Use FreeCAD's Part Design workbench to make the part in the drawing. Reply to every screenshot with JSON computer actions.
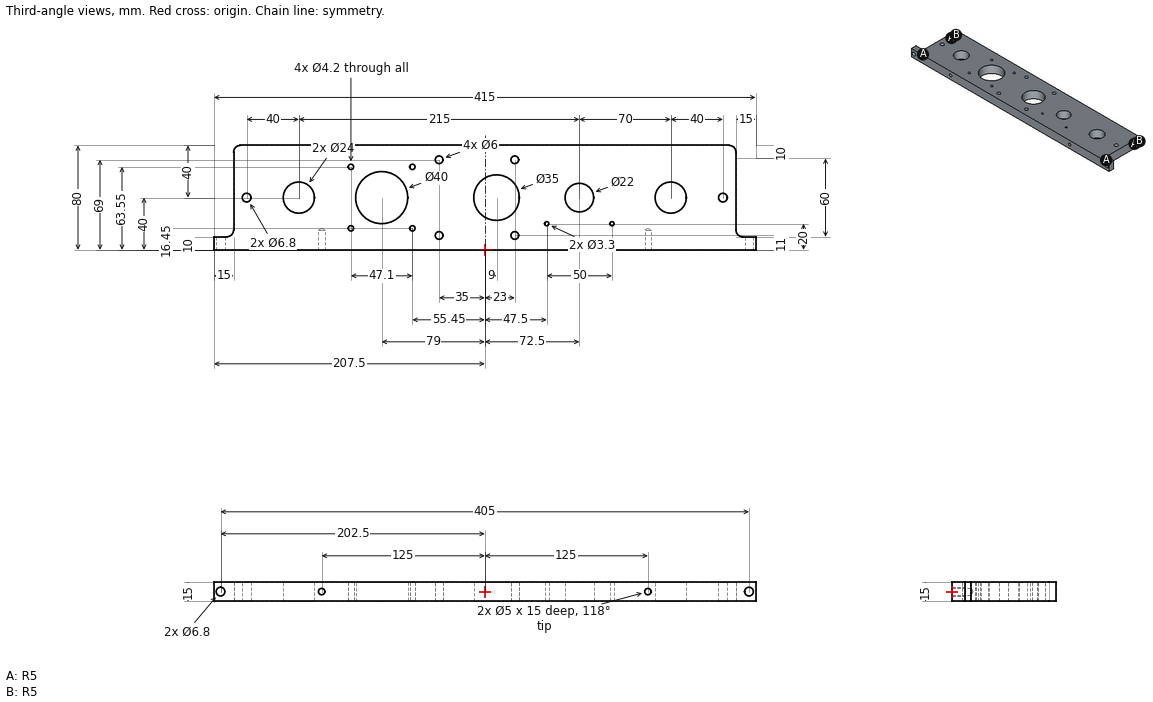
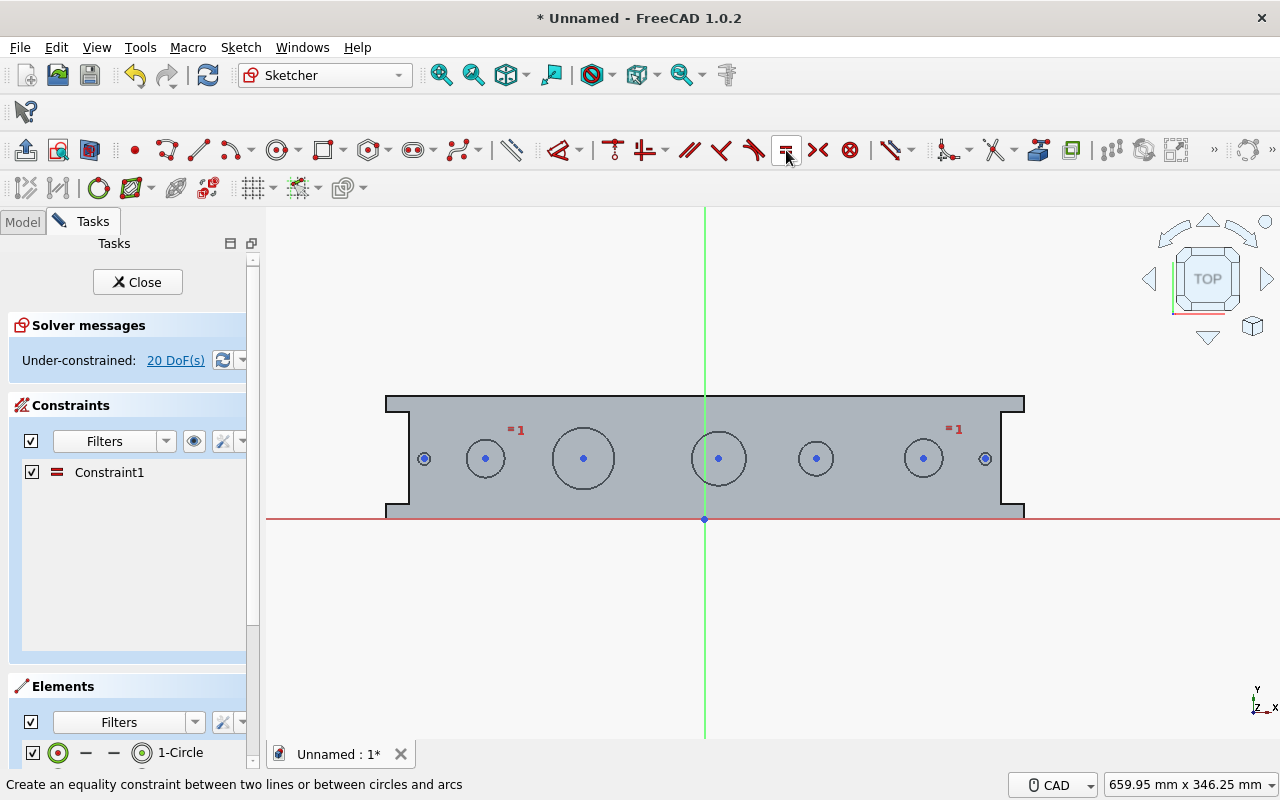
{"action": "scroll", "coordinate": [424, 453], "scroll_direction": "up", "scroll_amount": 5}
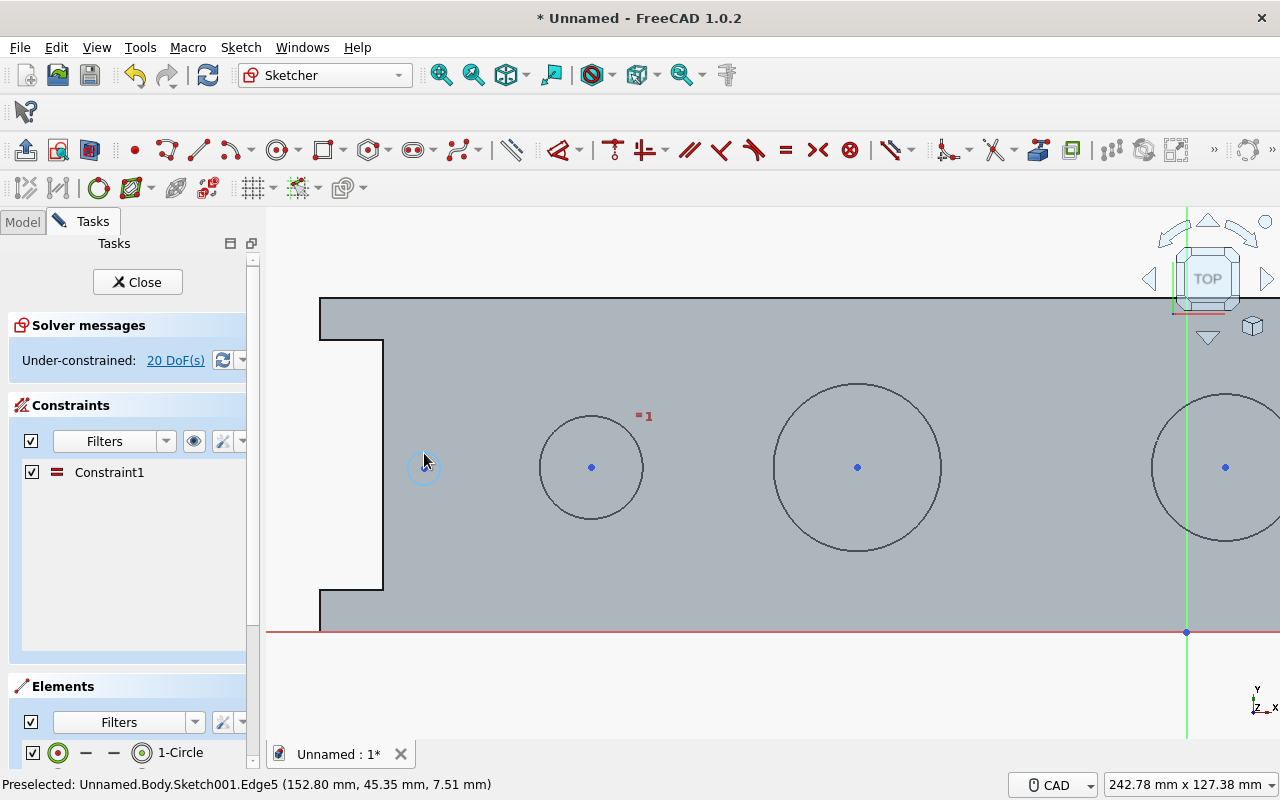
{"action": "left_click", "coordinate": [424, 452]}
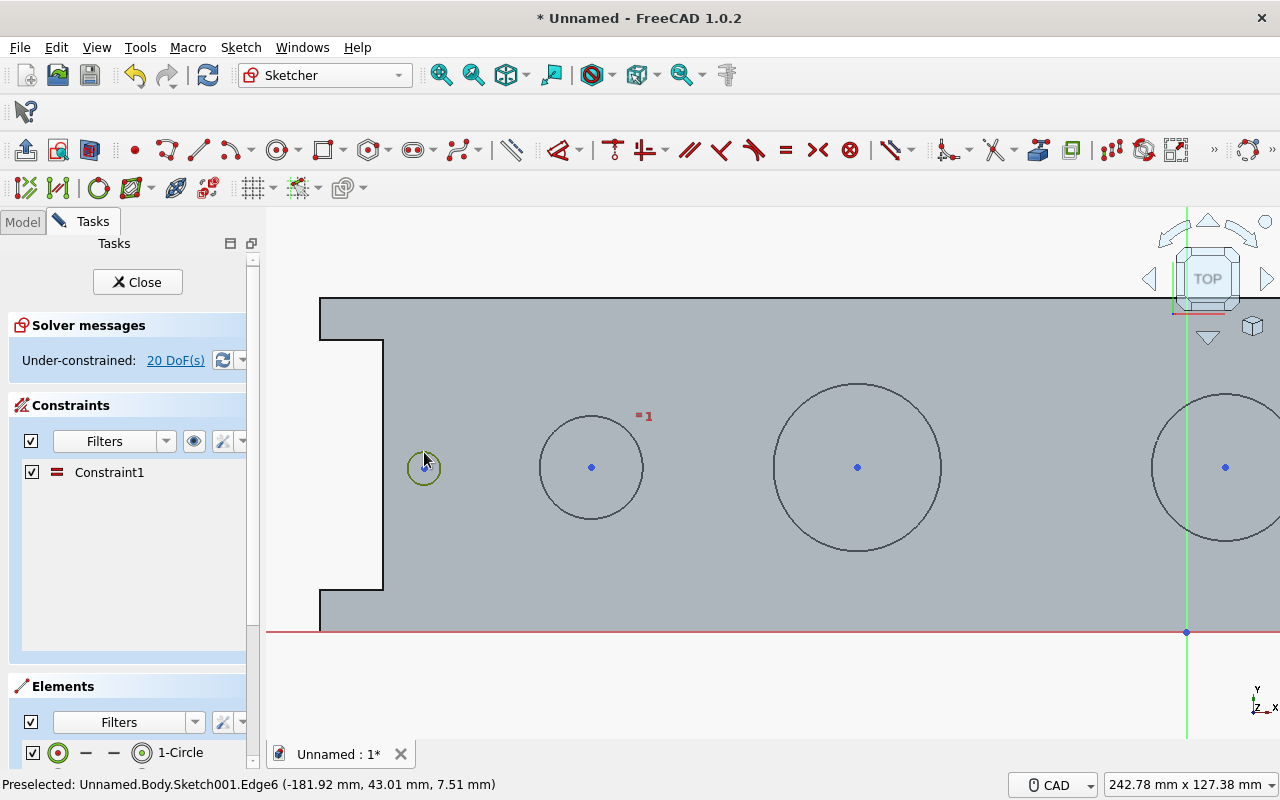
{"action": "scroll", "coordinate": [424, 453], "scroll_direction": "down", "scroll_amount": 5}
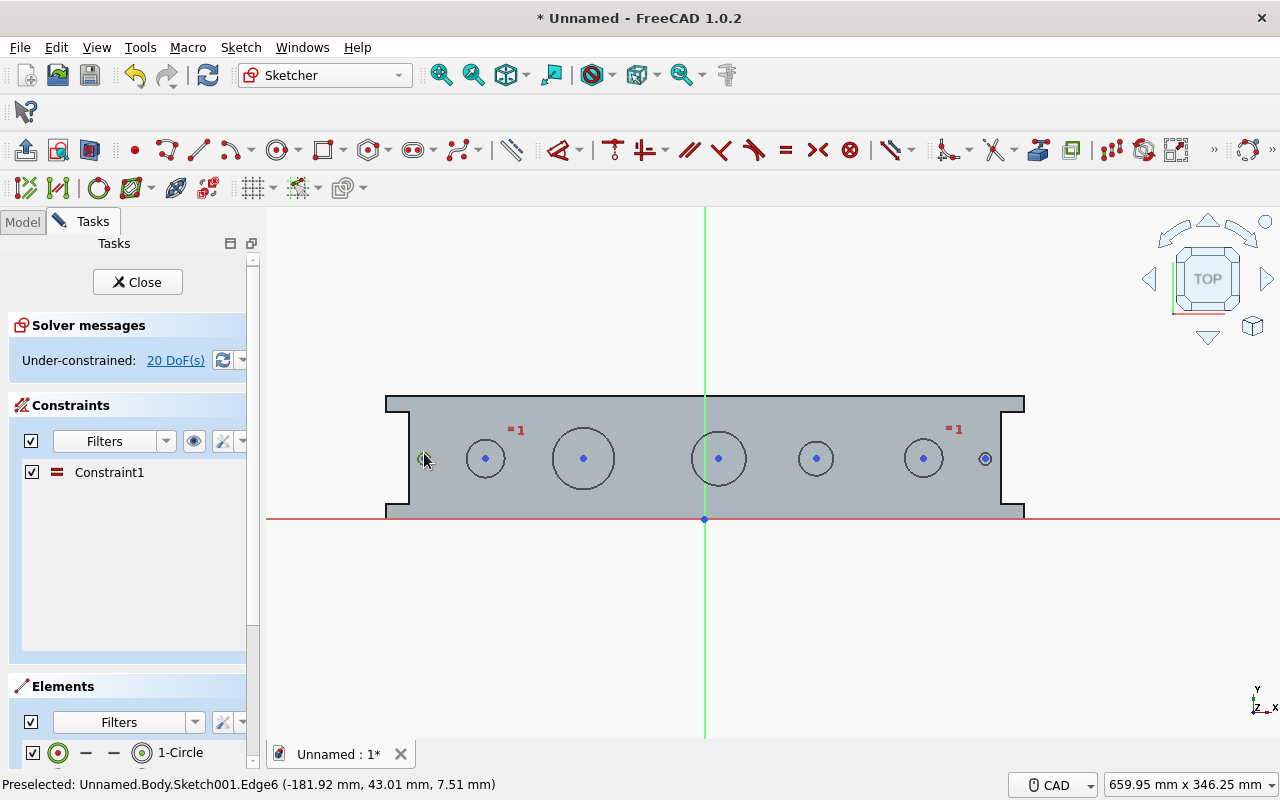
{"action": "scroll", "coordinate": [989, 455], "scroll_direction": "up", "scroll_amount": 5}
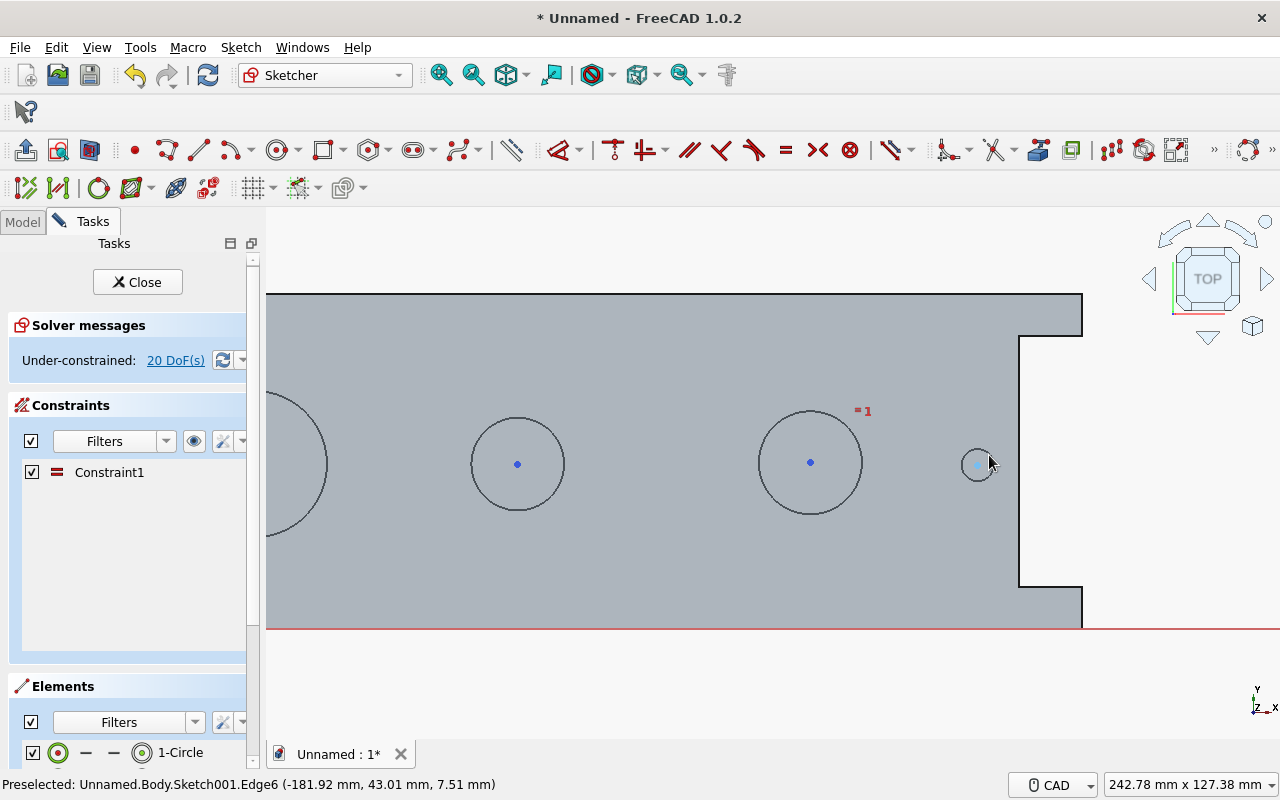
{"action": "left_click", "coordinate": [989, 454]}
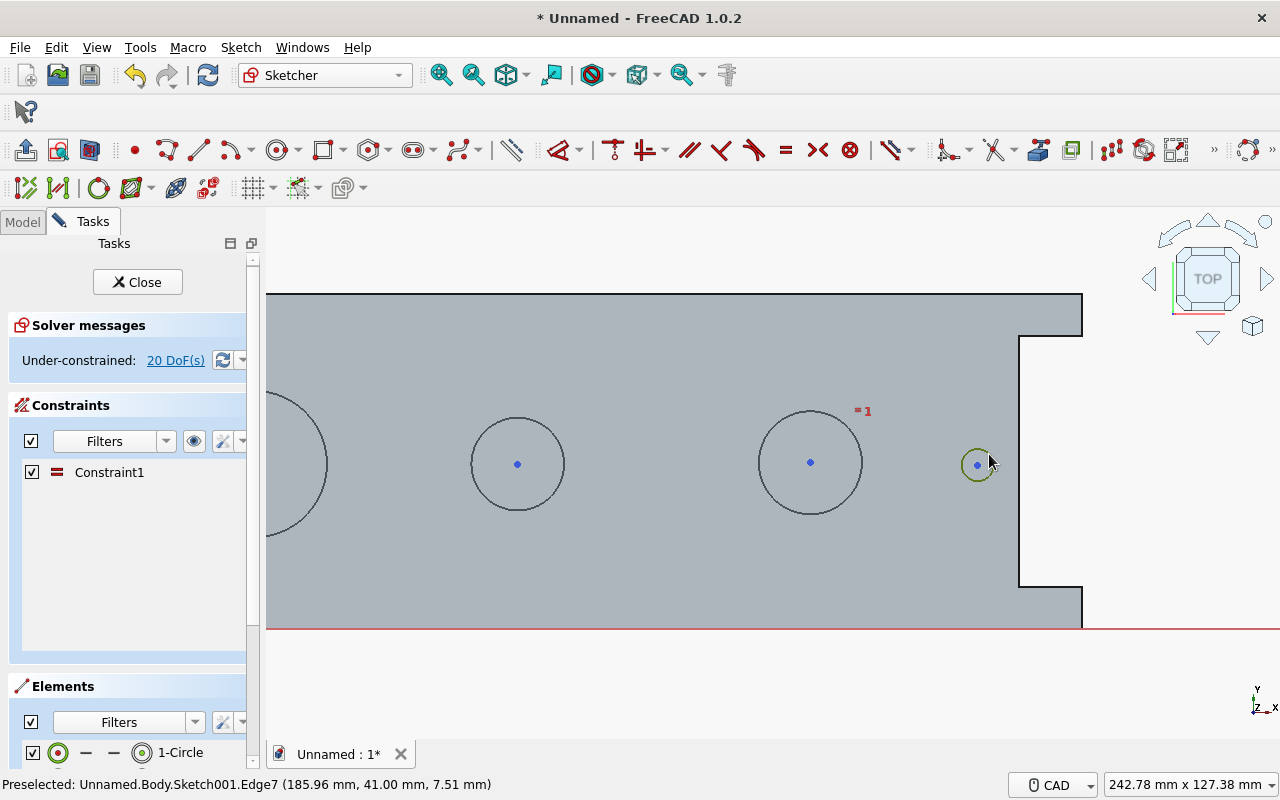
{"action": "left_click", "coordinate": [786, 150]}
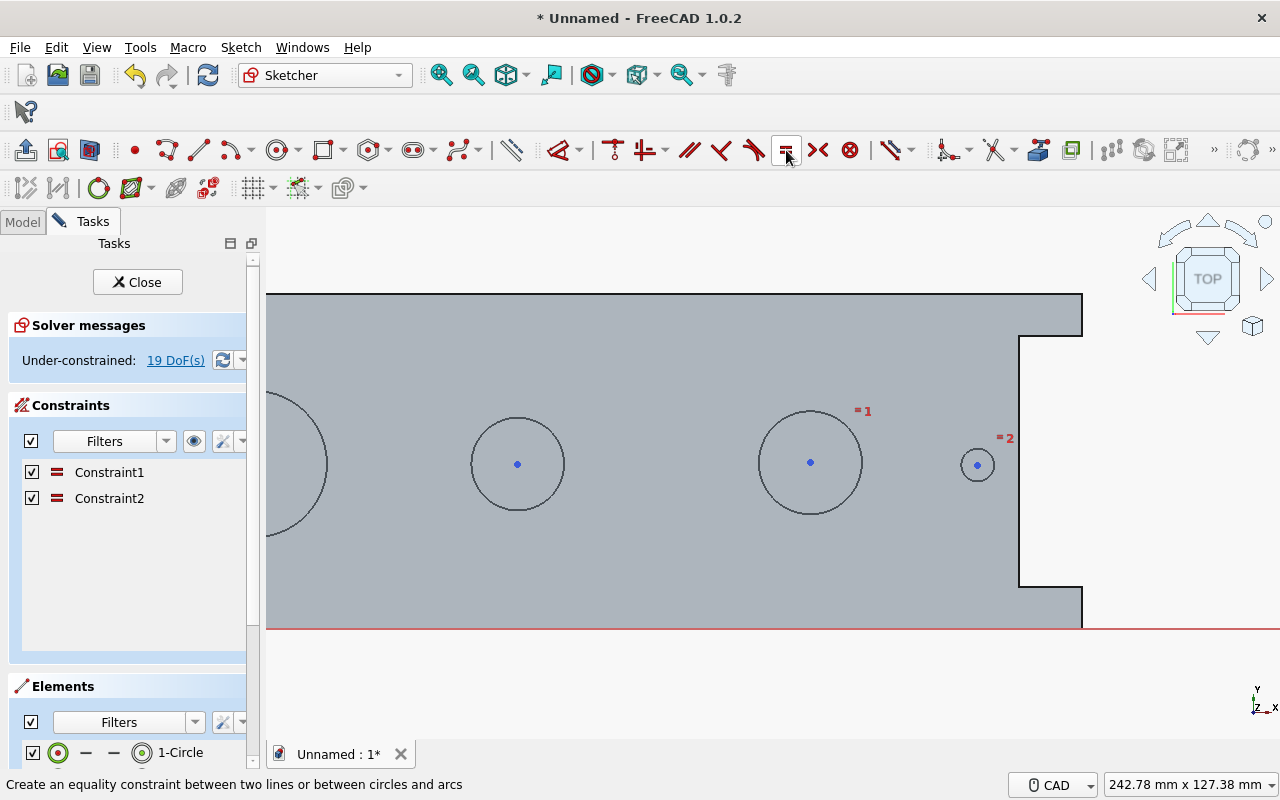
{"action": "scroll", "coordinate": [989, 455], "scroll_direction": "down", "scroll_amount": 5}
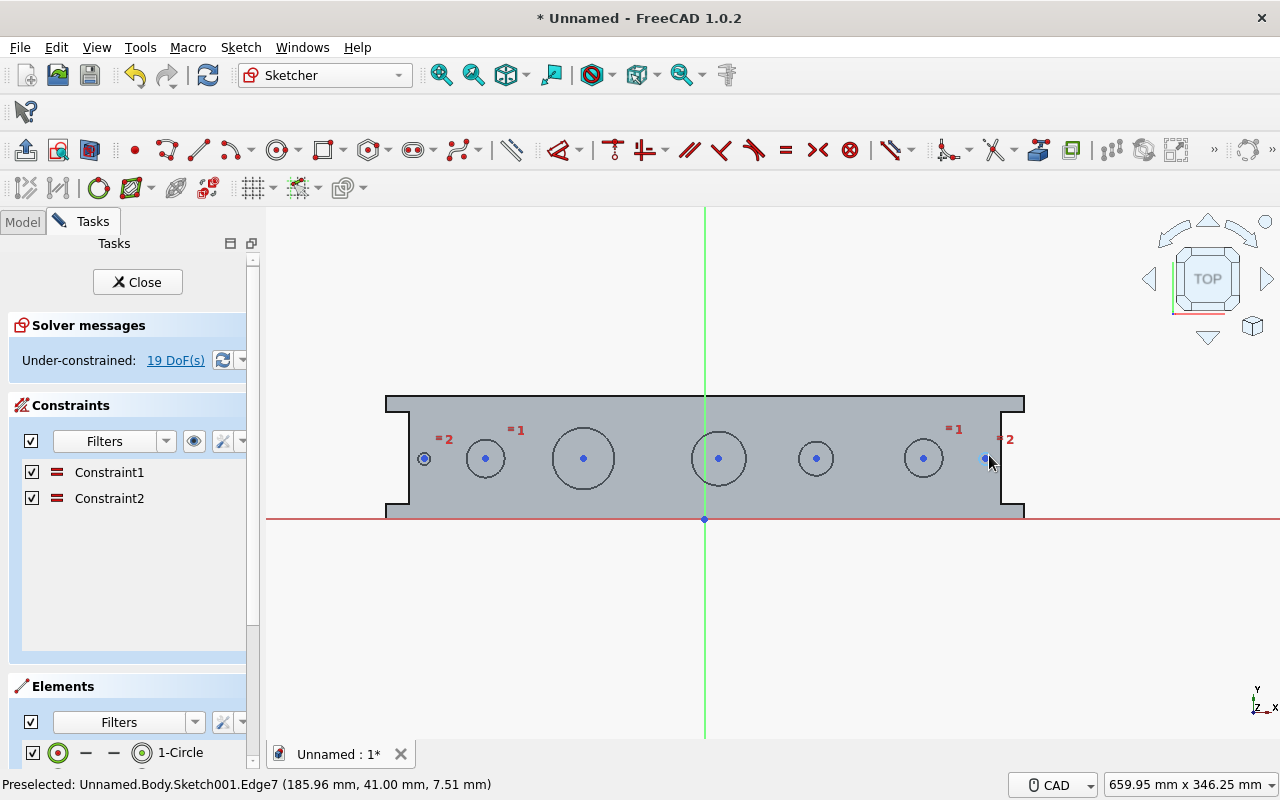
{"action": "left_click", "coordinate": [486, 459]}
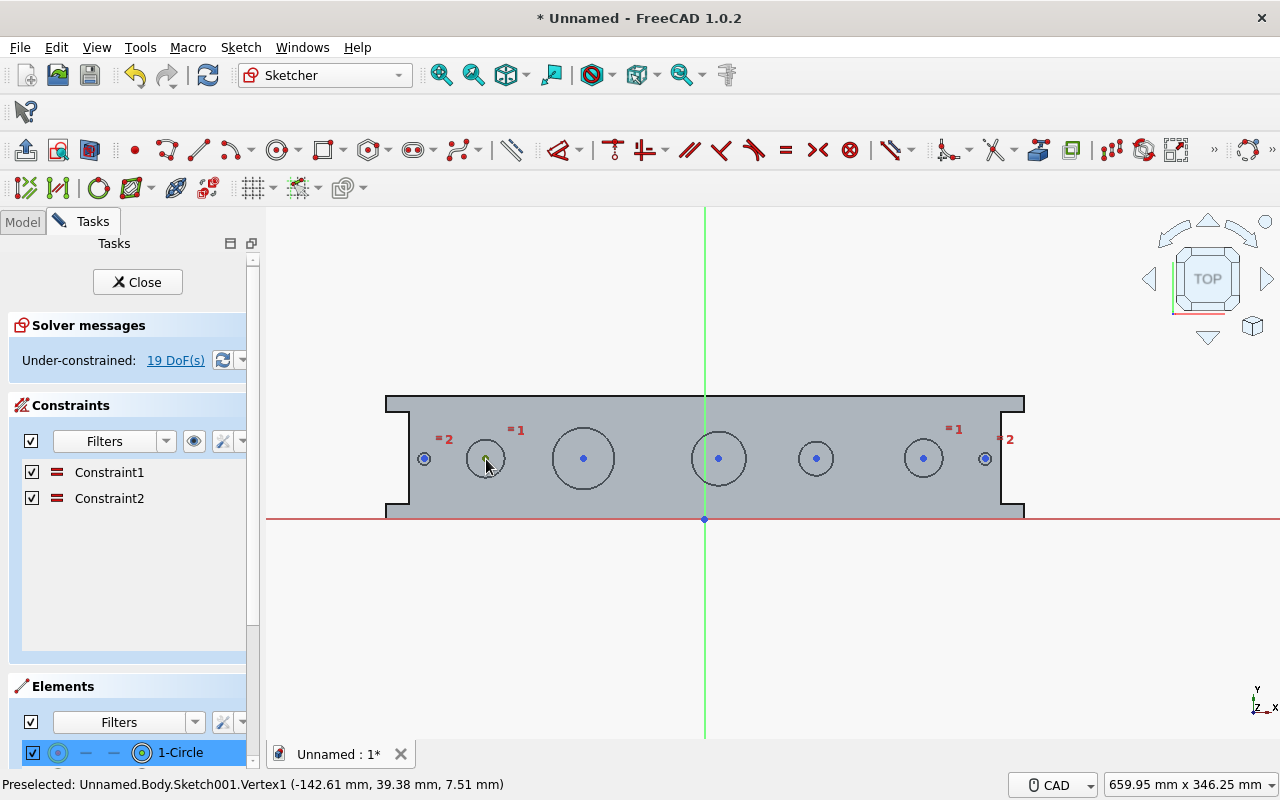
{"action": "left_click", "coordinate": [719, 459]}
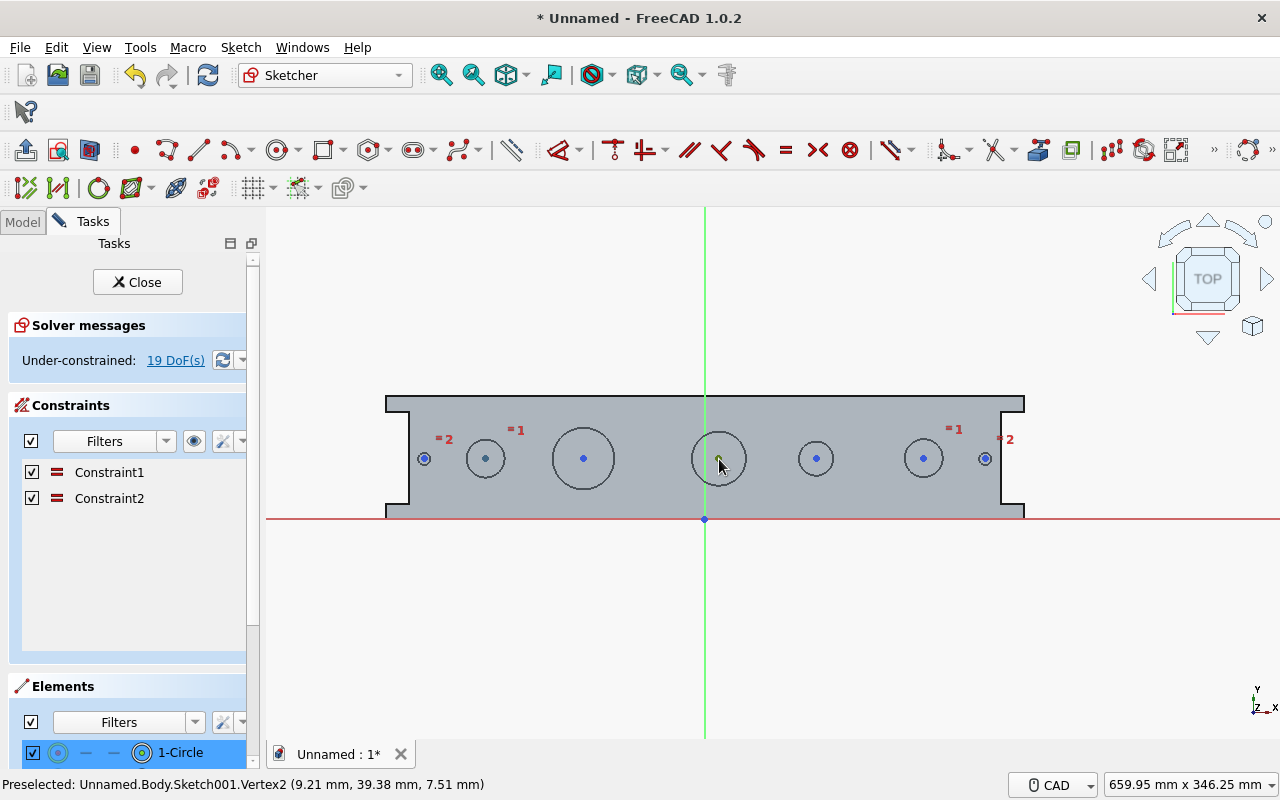
{"action": "left_click", "coordinate": [668, 150]}